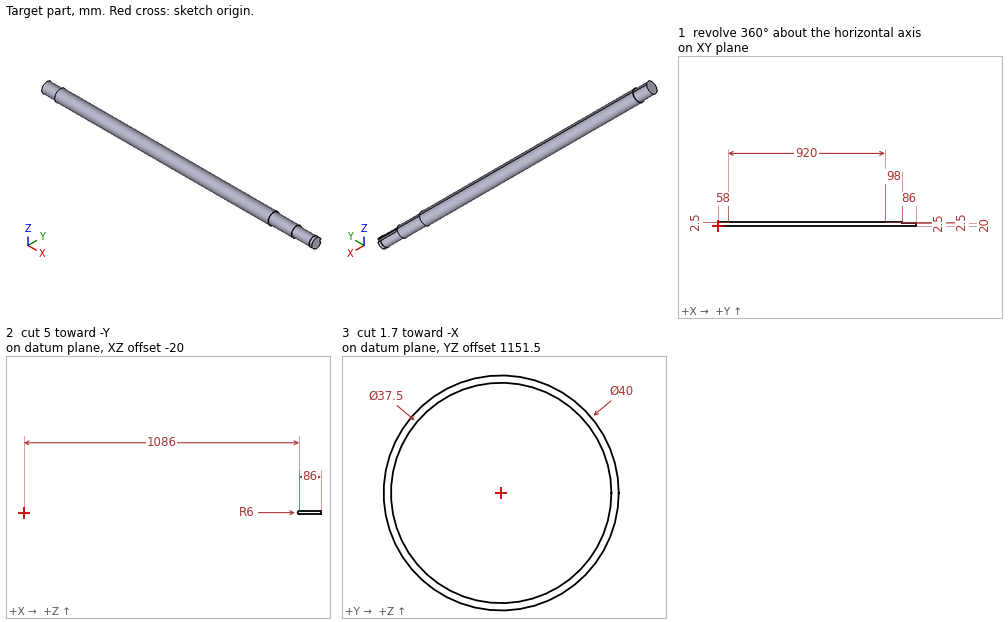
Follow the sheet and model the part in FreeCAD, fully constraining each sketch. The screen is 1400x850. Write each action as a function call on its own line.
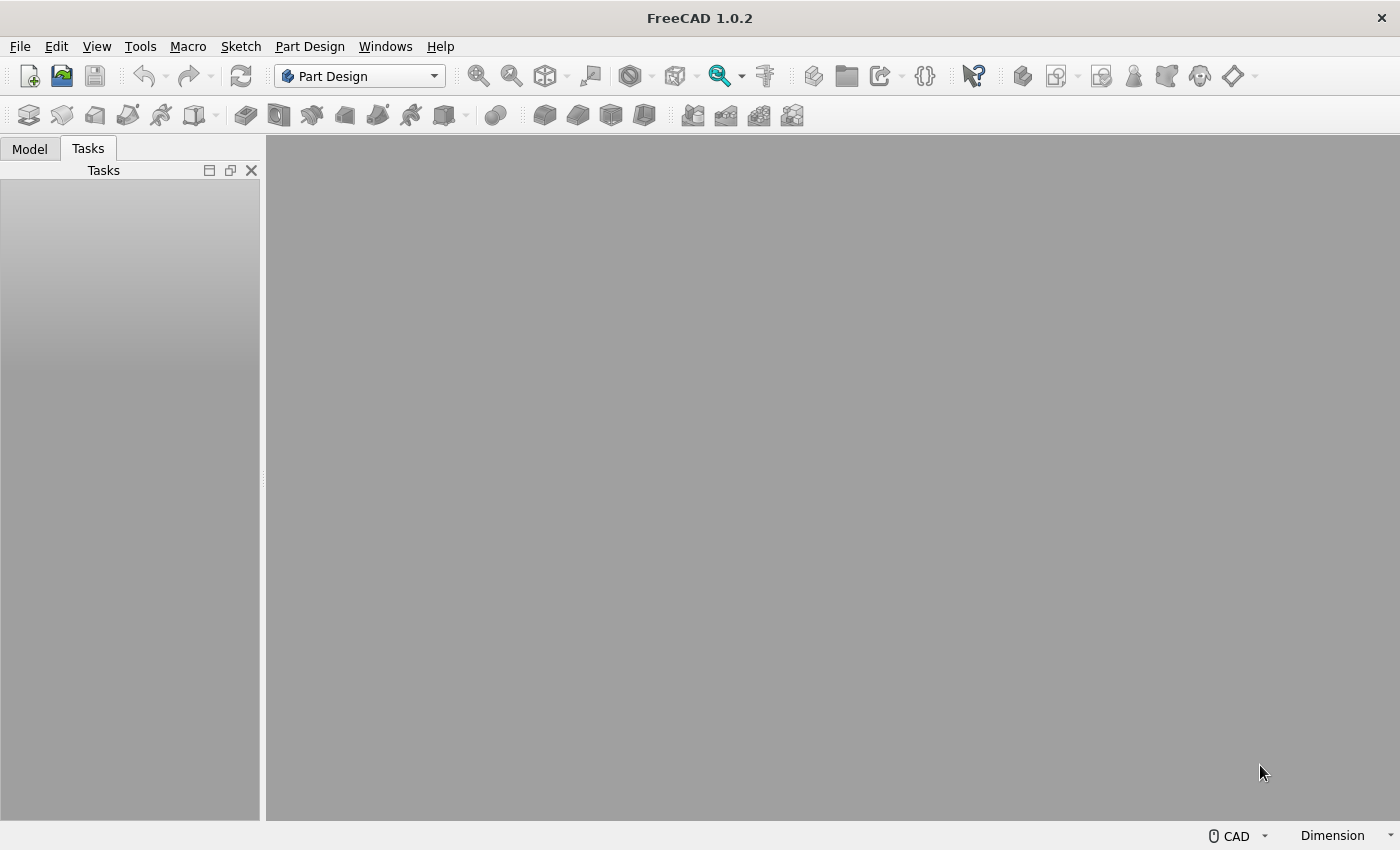
click(29, 76)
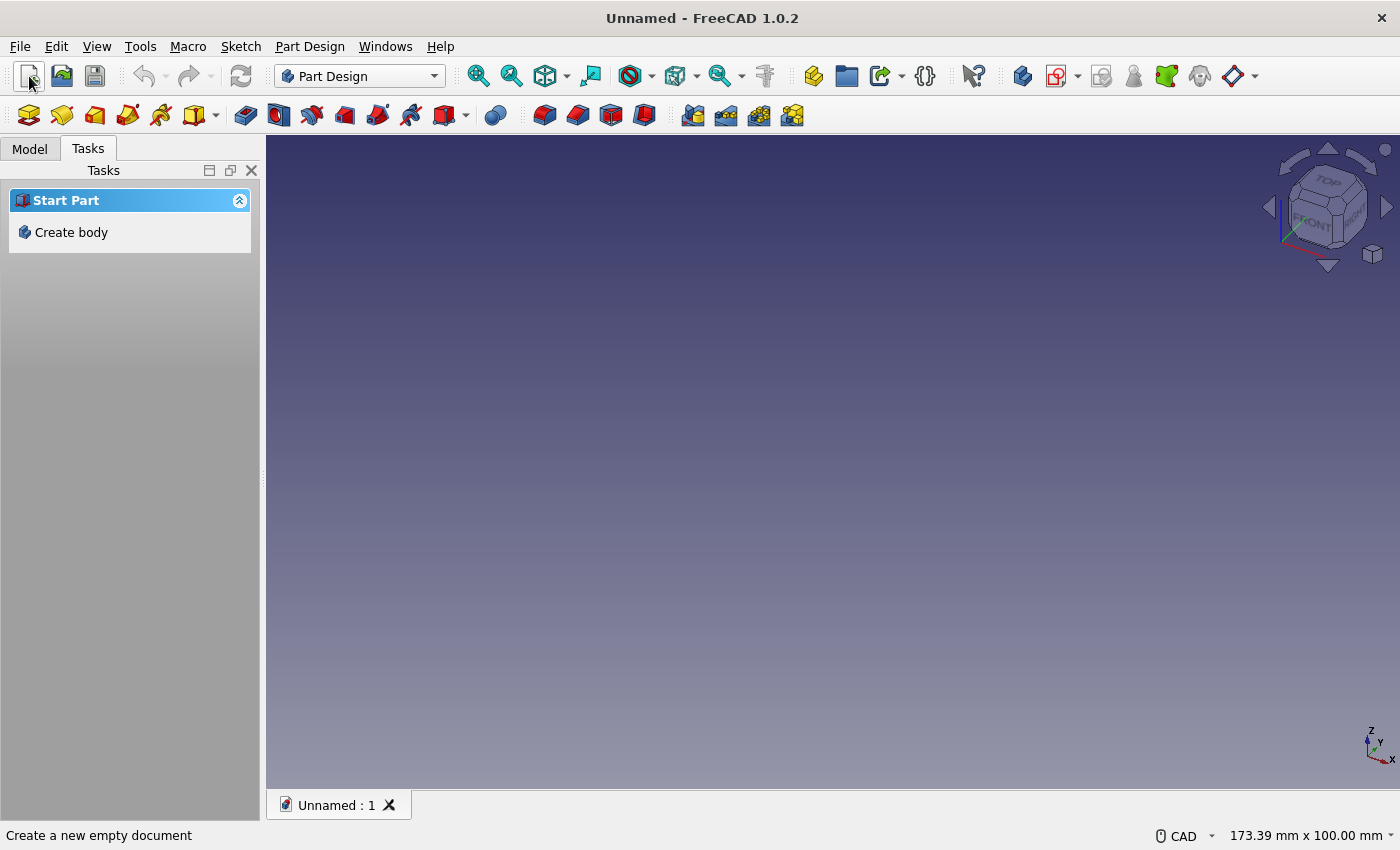
click(1056, 76)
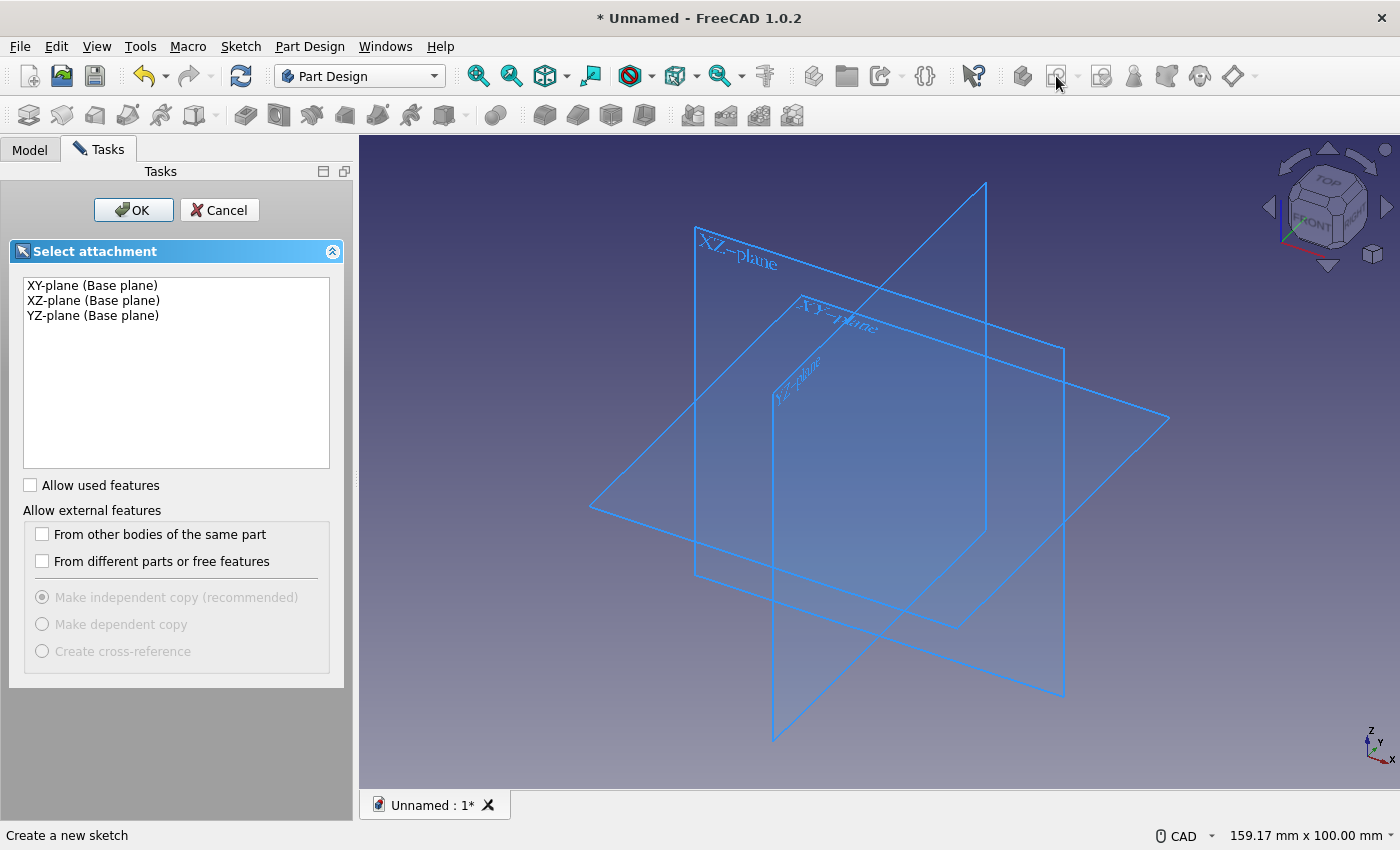
click(84, 286)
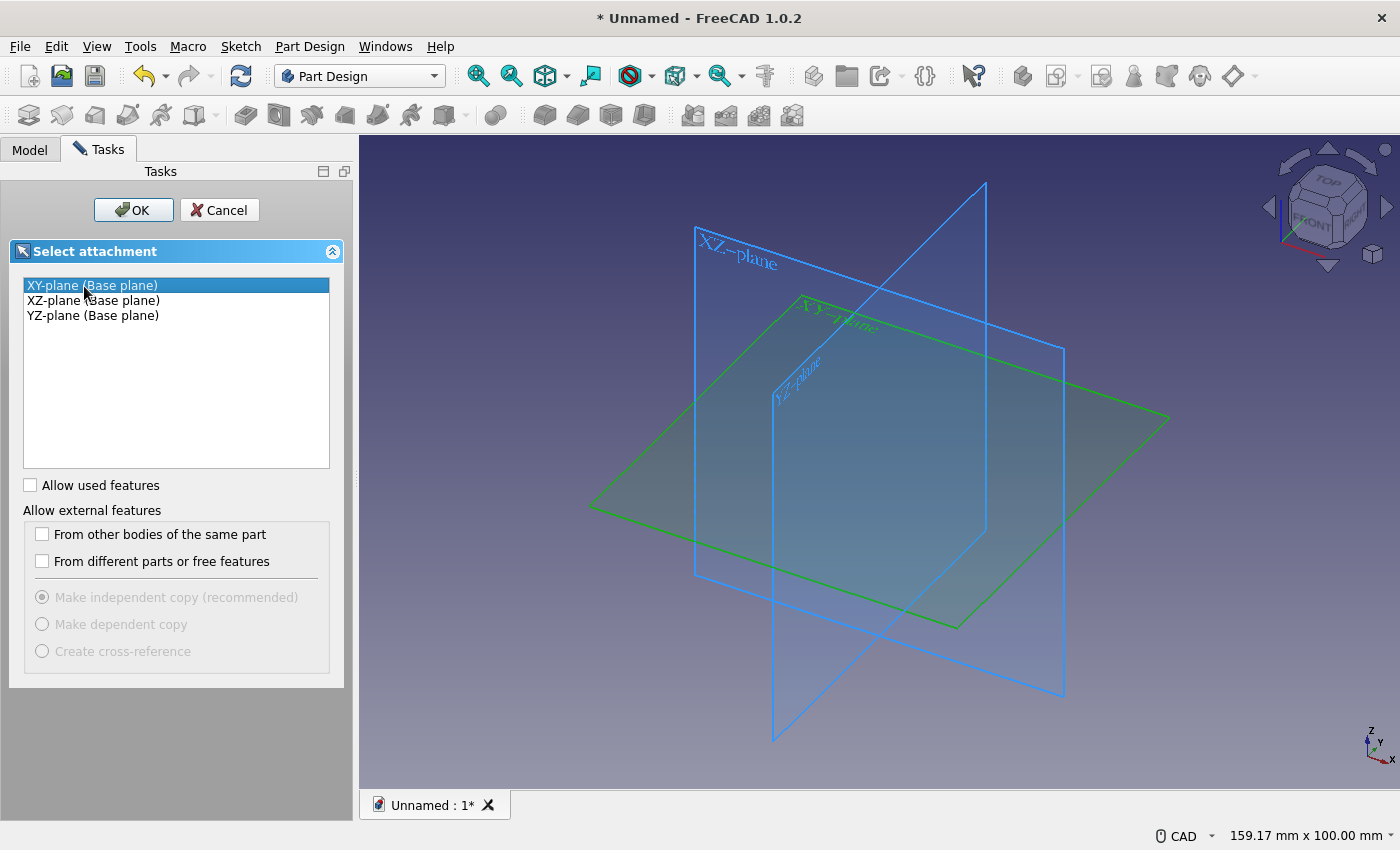
click(134, 210)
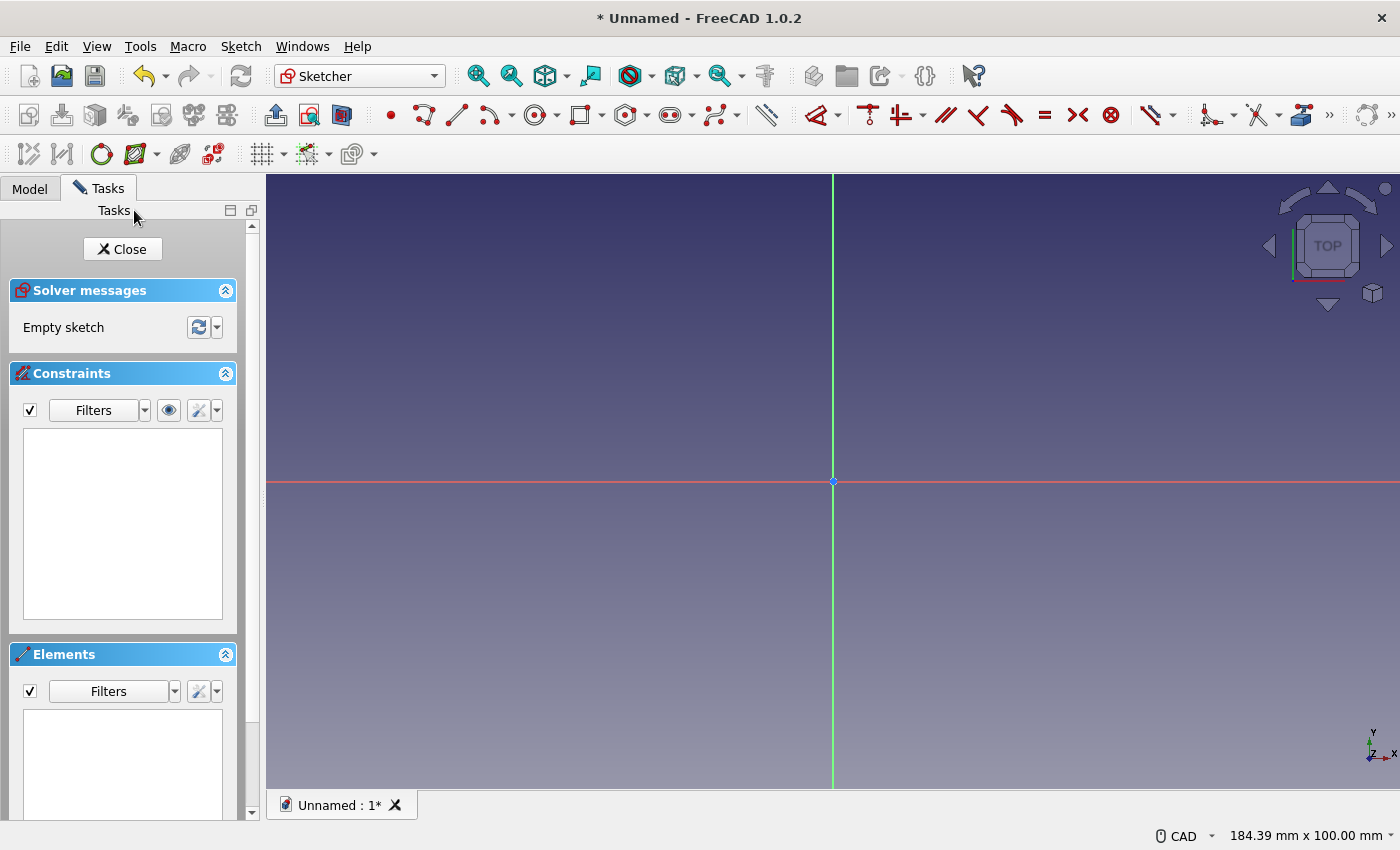
scroll(401, 489, down, 12)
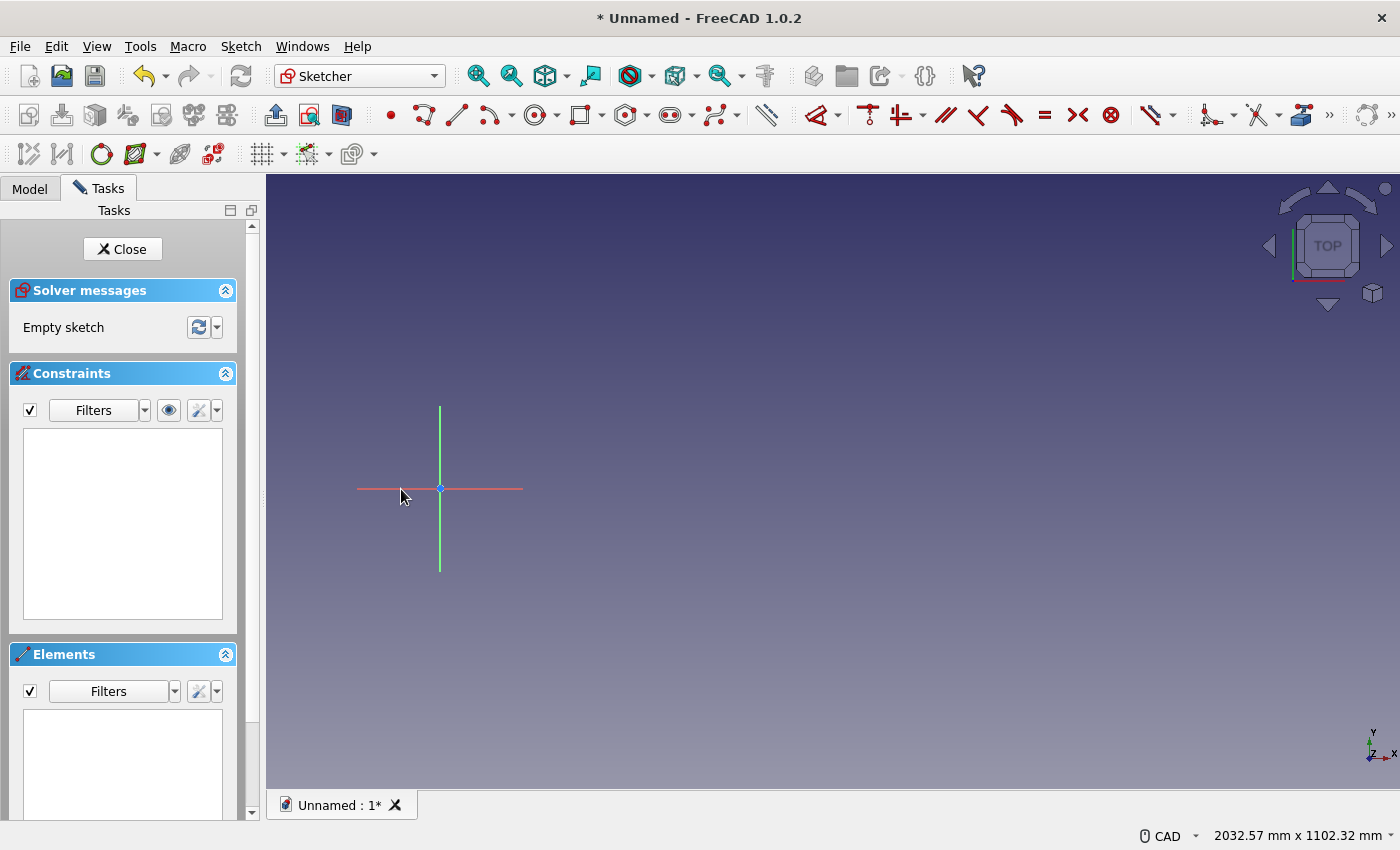
click(424, 116)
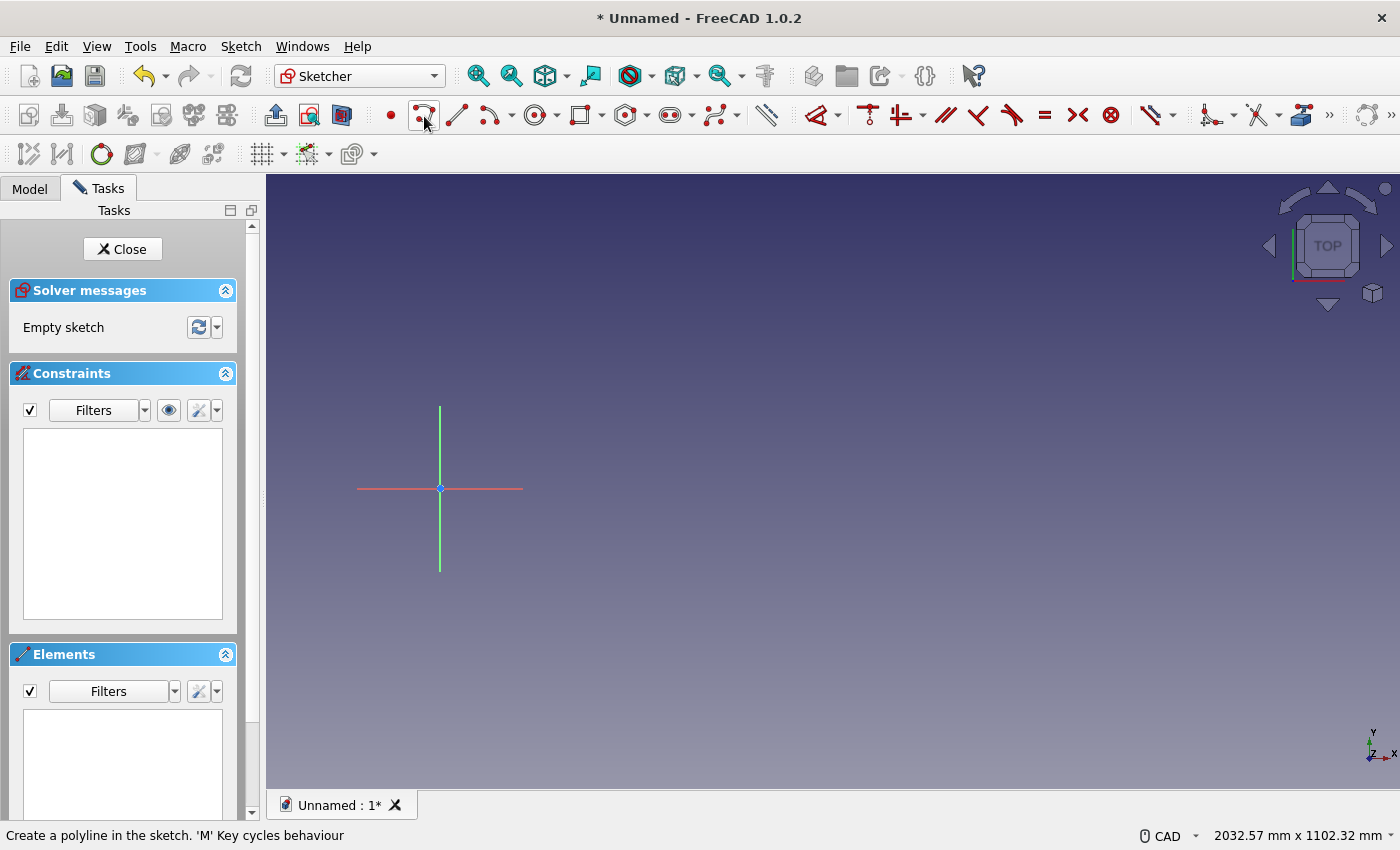
click(440, 489)
click(1089, 480)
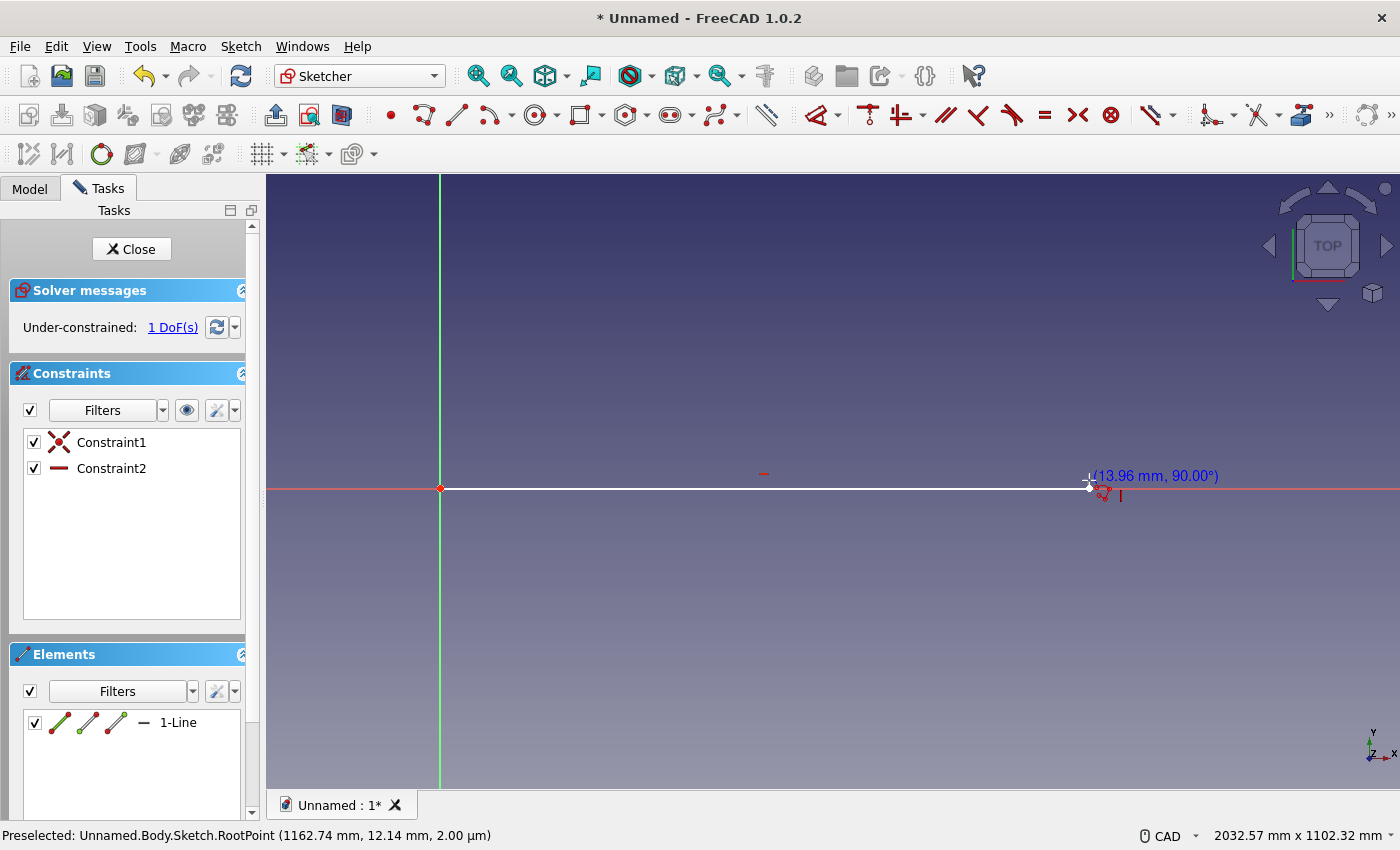
scroll(1089, 478, up, 2)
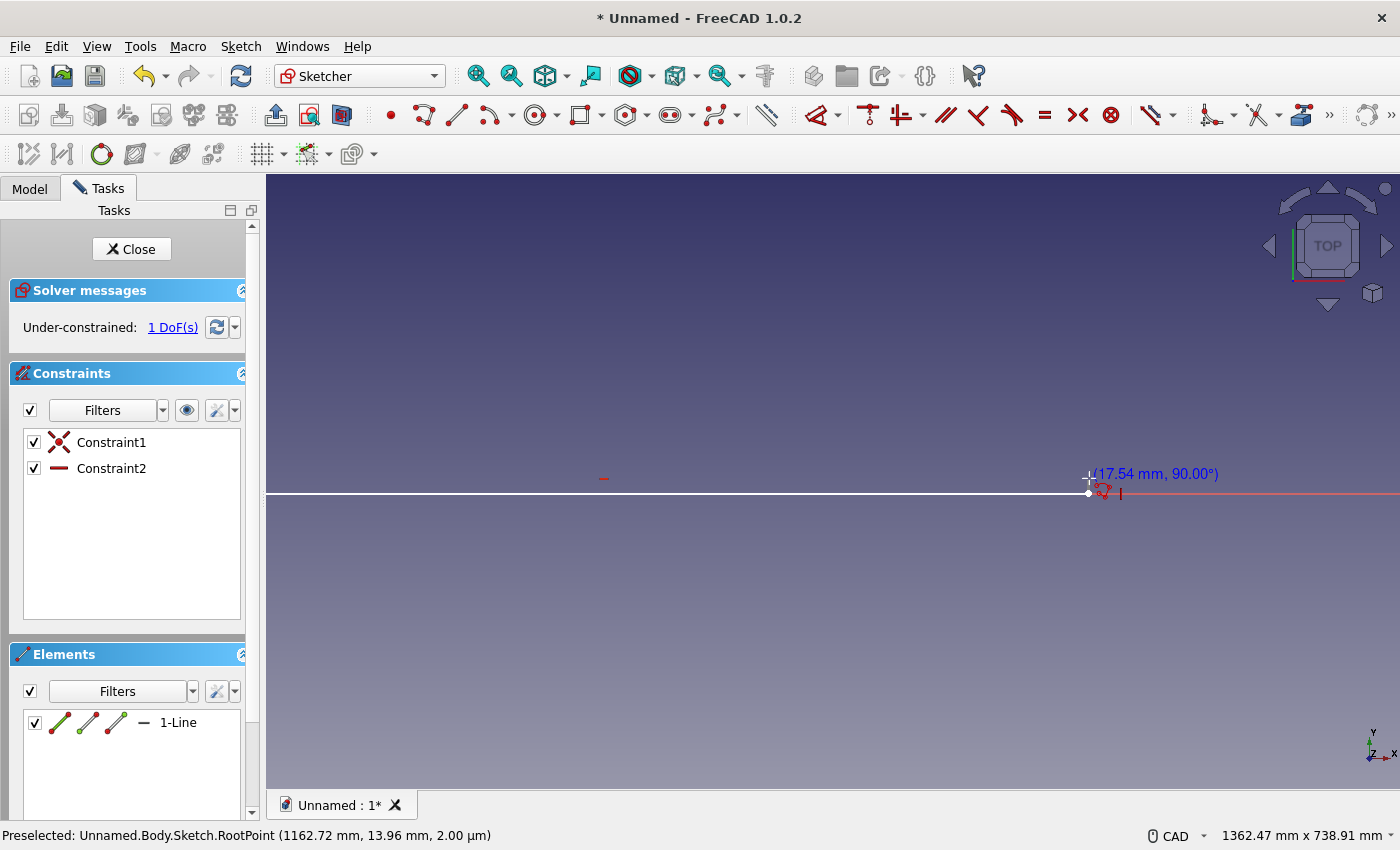
click(1089, 477)
click(1016, 477)